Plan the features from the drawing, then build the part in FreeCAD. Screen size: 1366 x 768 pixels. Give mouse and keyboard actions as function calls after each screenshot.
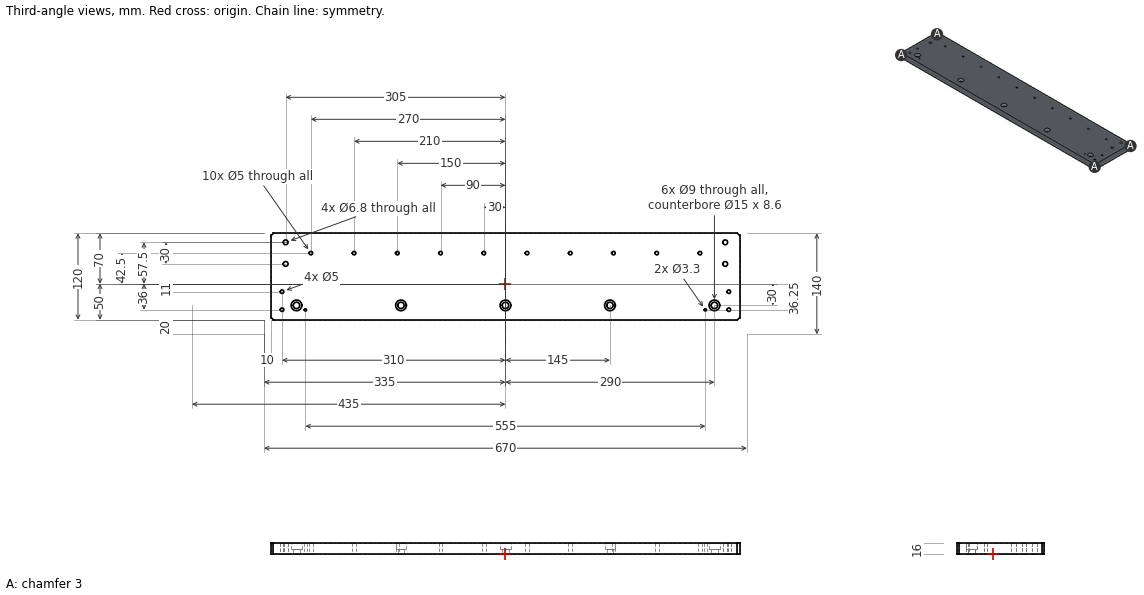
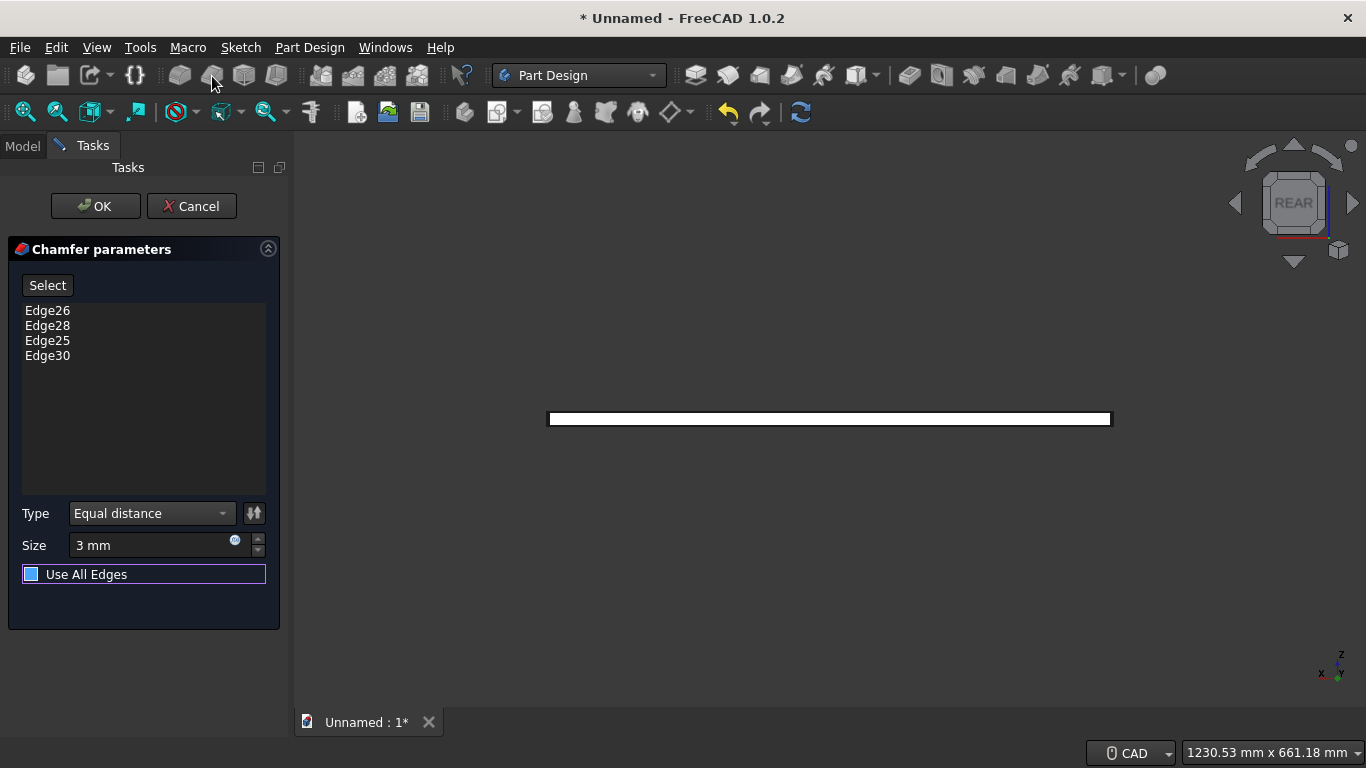
click(96, 206)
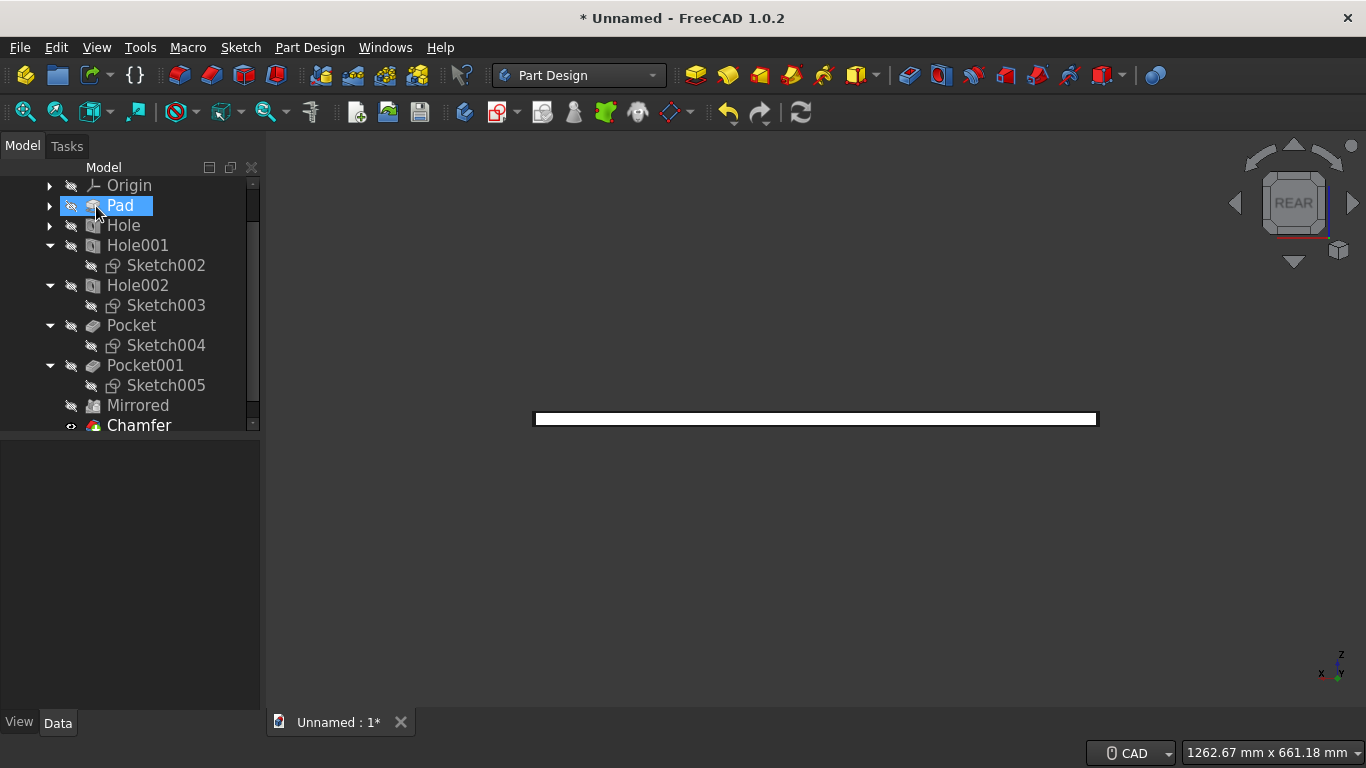
key(0)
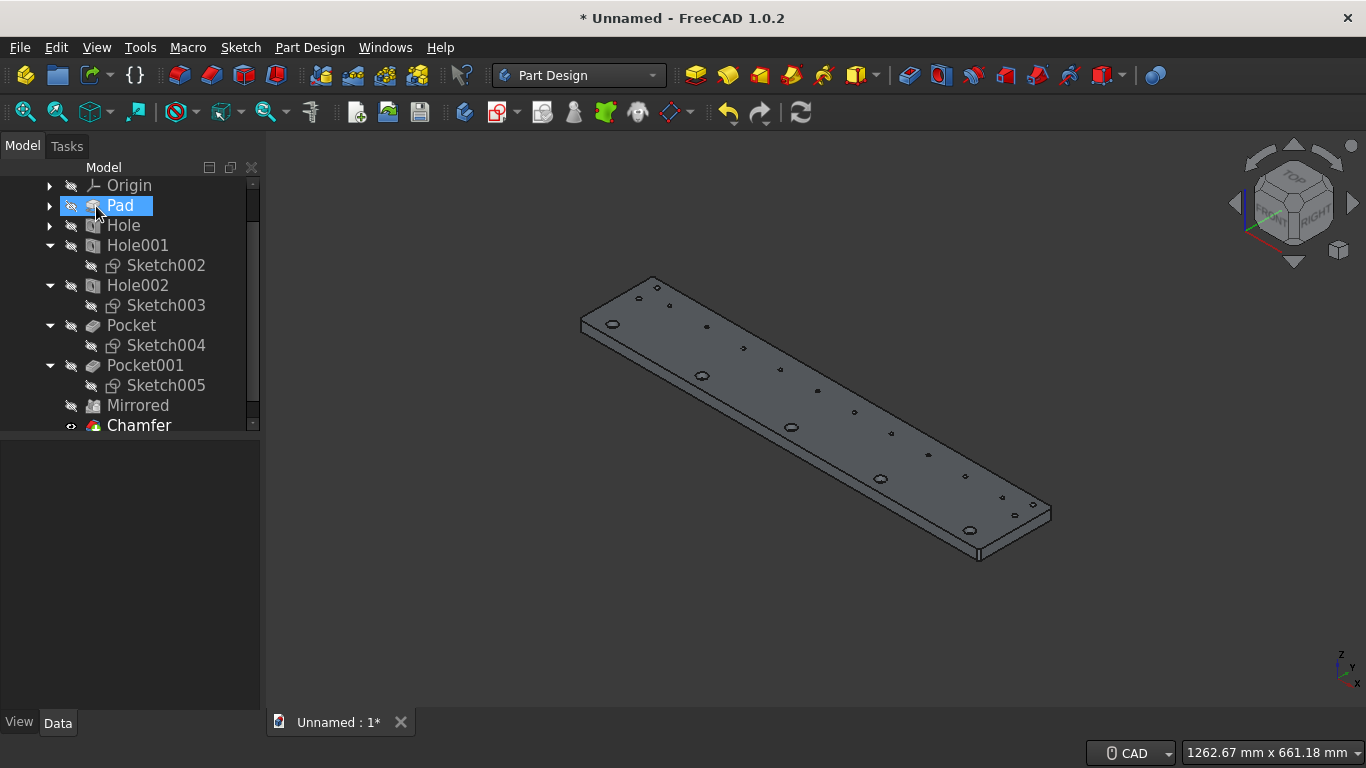
click(863, 451)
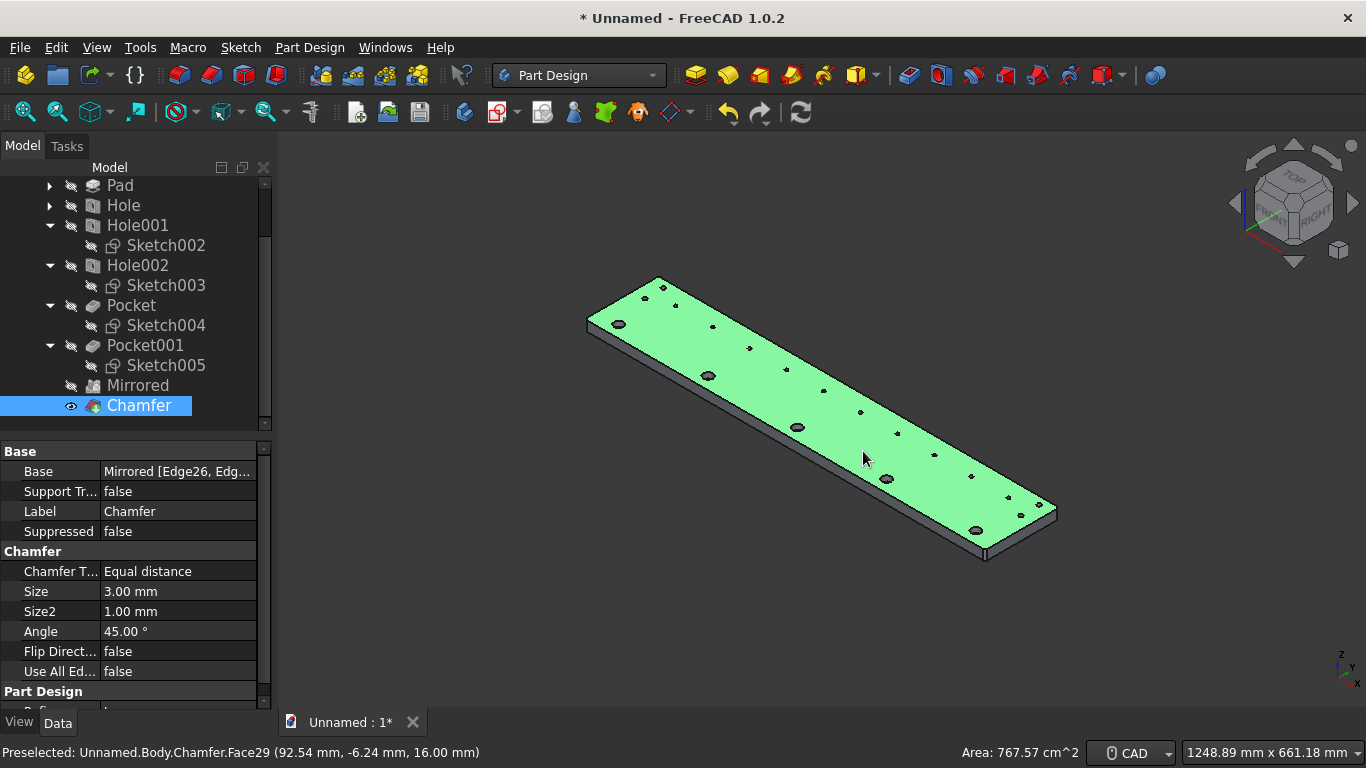
click(498, 112)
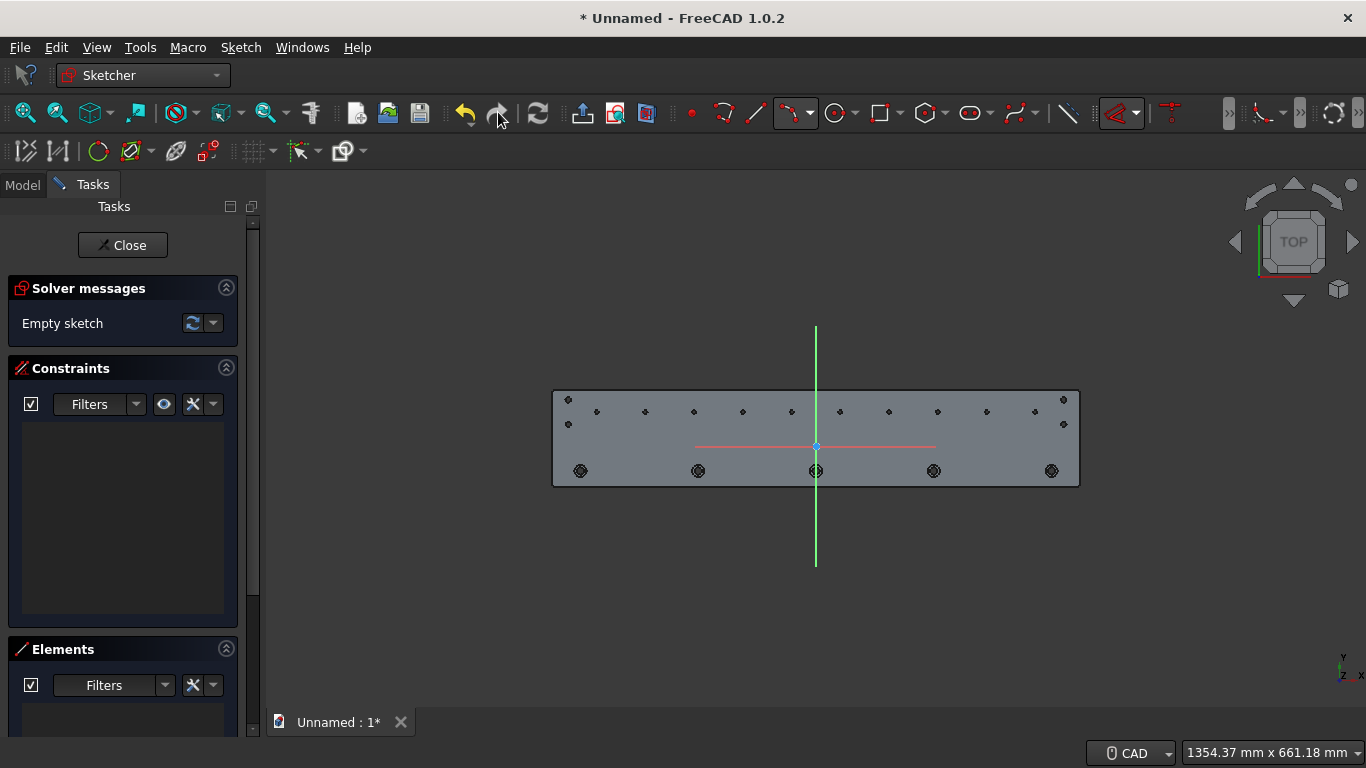
click(836, 114)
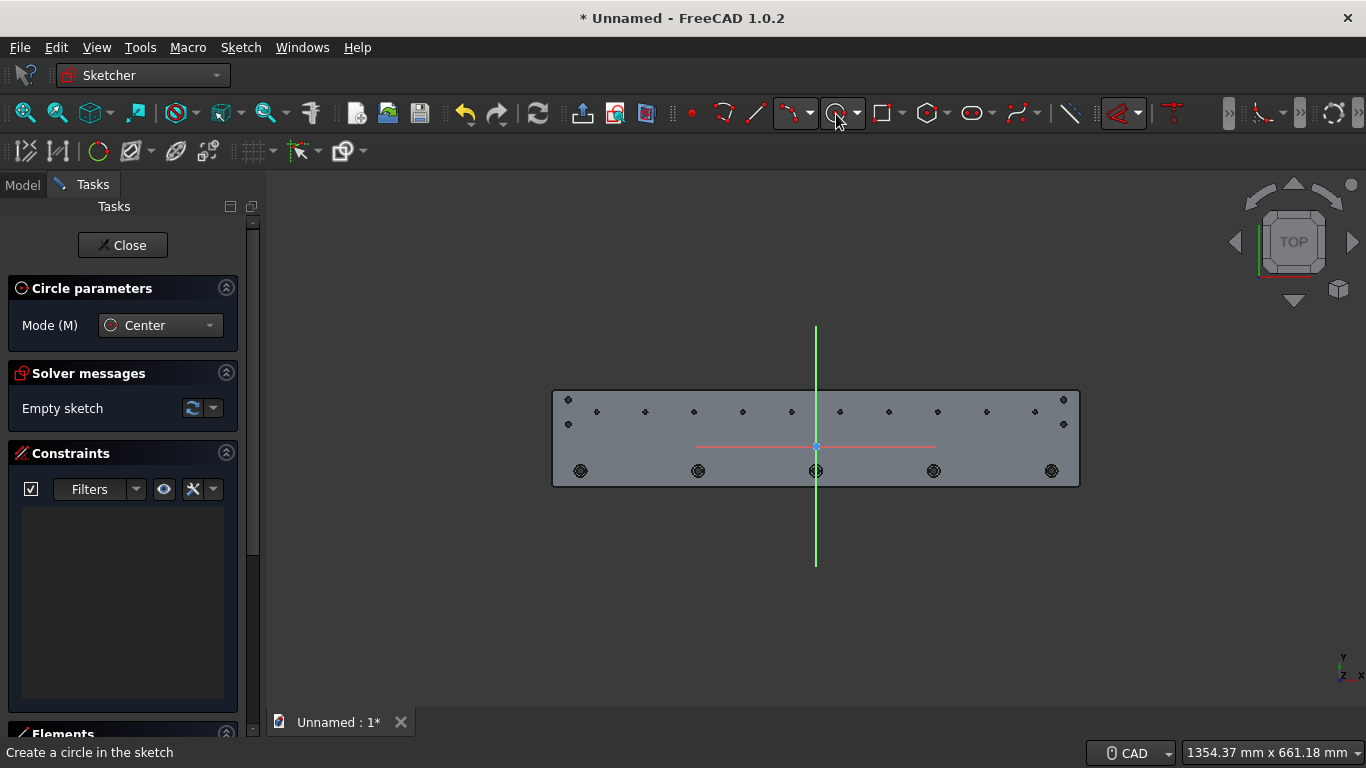
scroll(564, 456, up, 13)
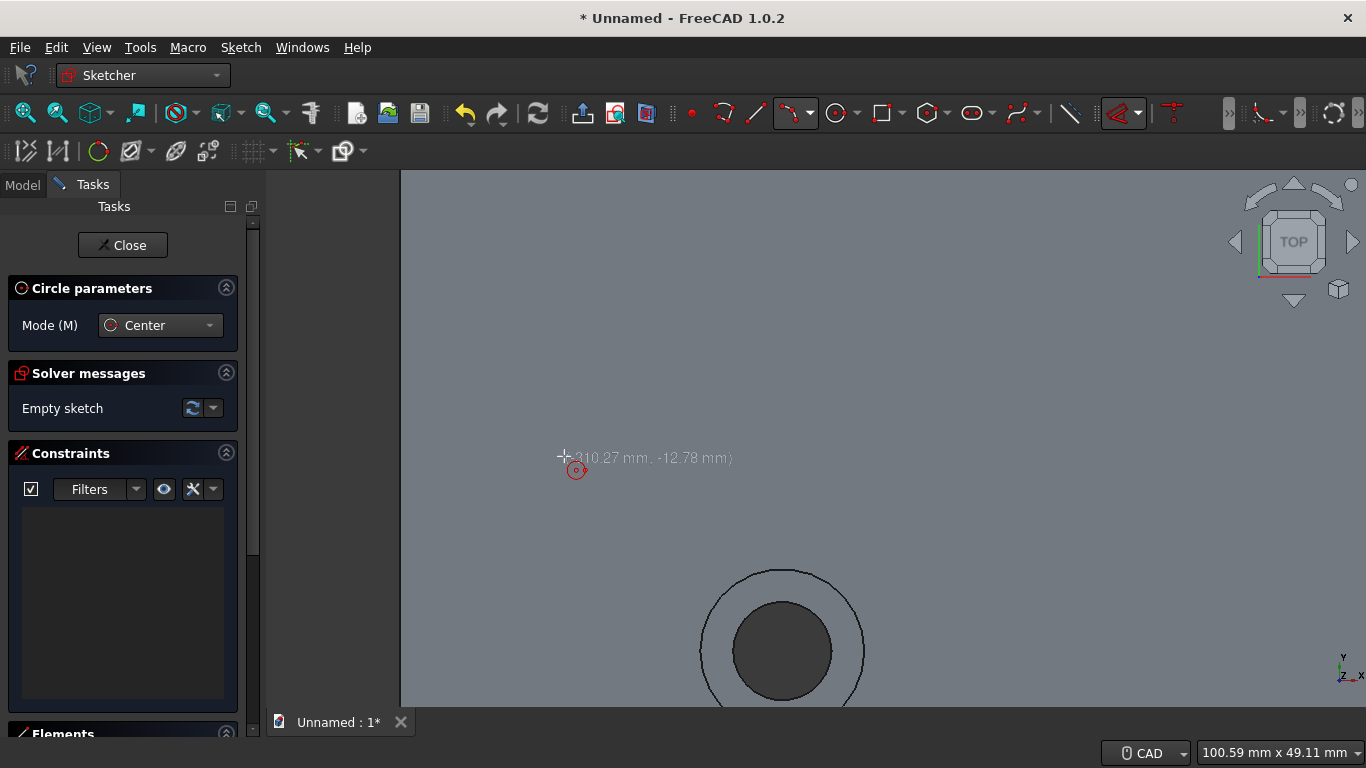
scroll(428, 429, down, 12)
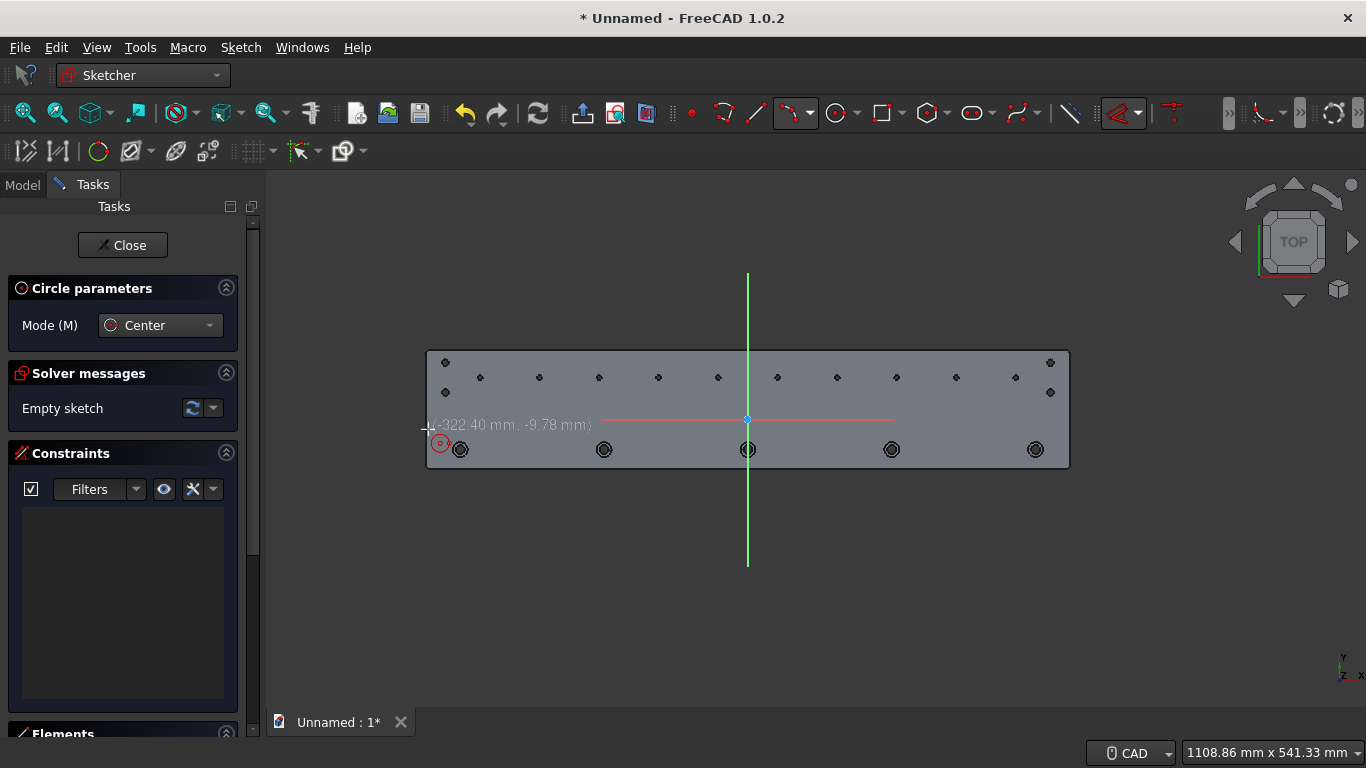
scroll(440, 431, up, 2)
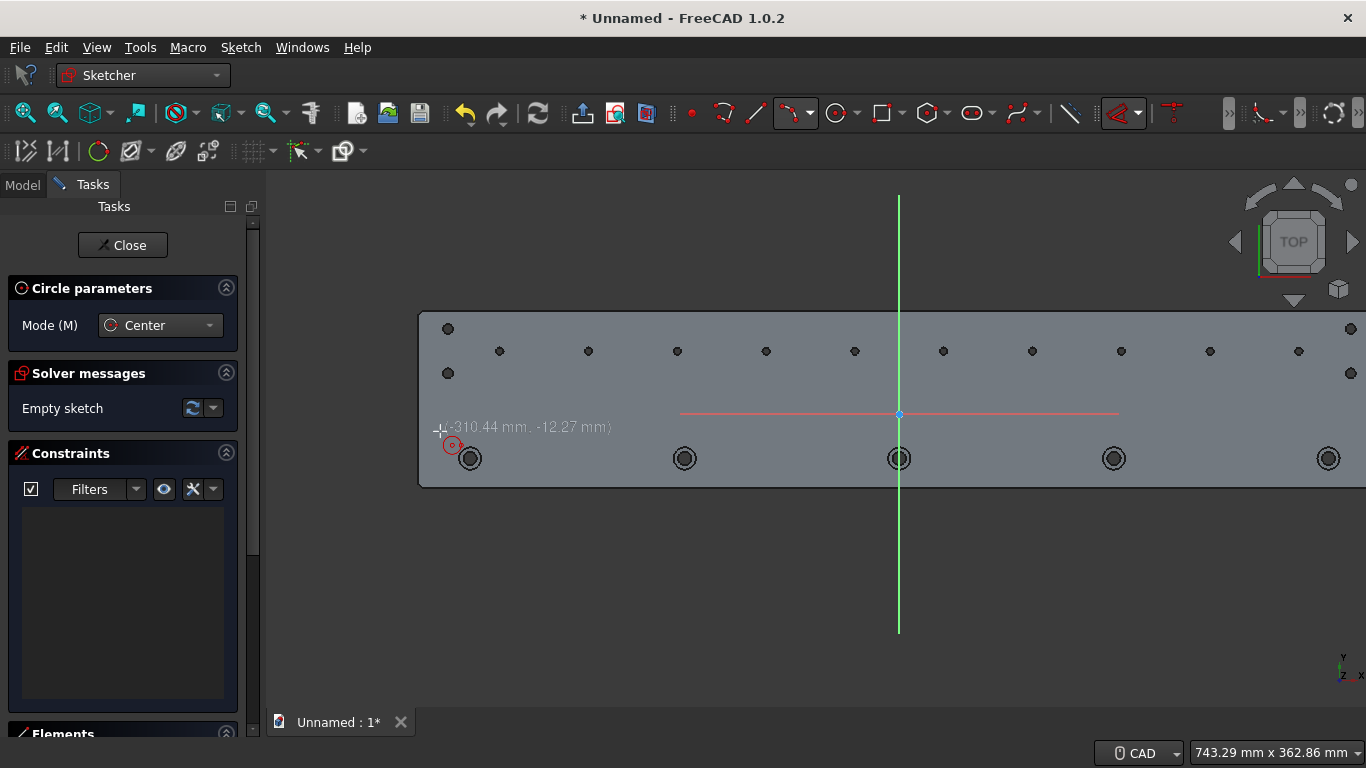
click(441, 430)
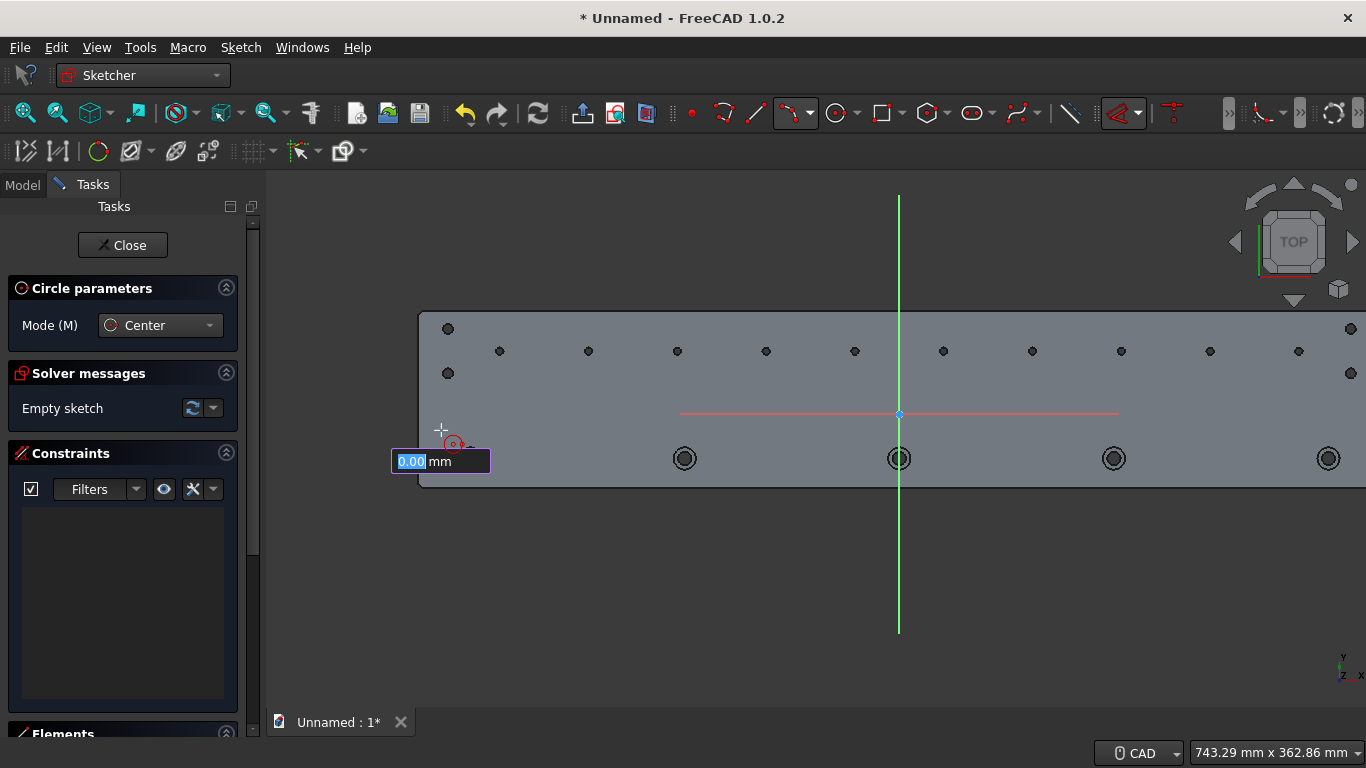
scroll(443, 433, up, 8)